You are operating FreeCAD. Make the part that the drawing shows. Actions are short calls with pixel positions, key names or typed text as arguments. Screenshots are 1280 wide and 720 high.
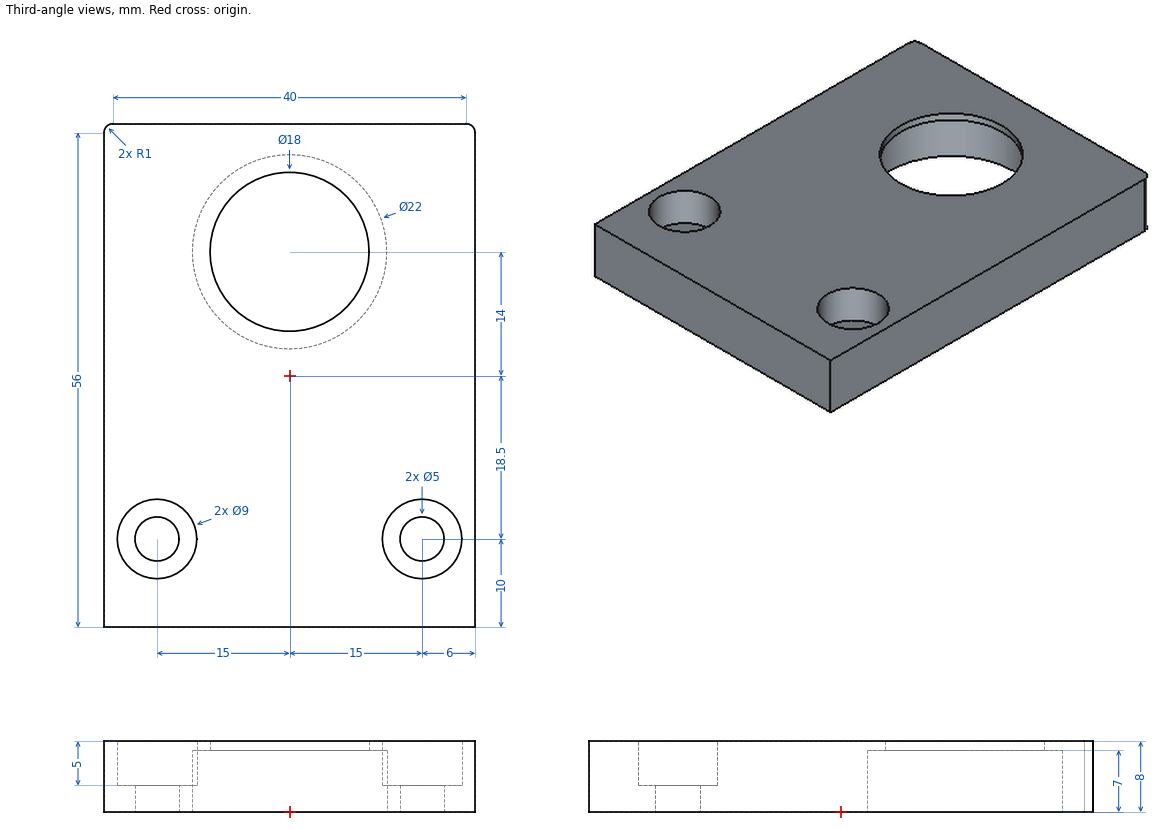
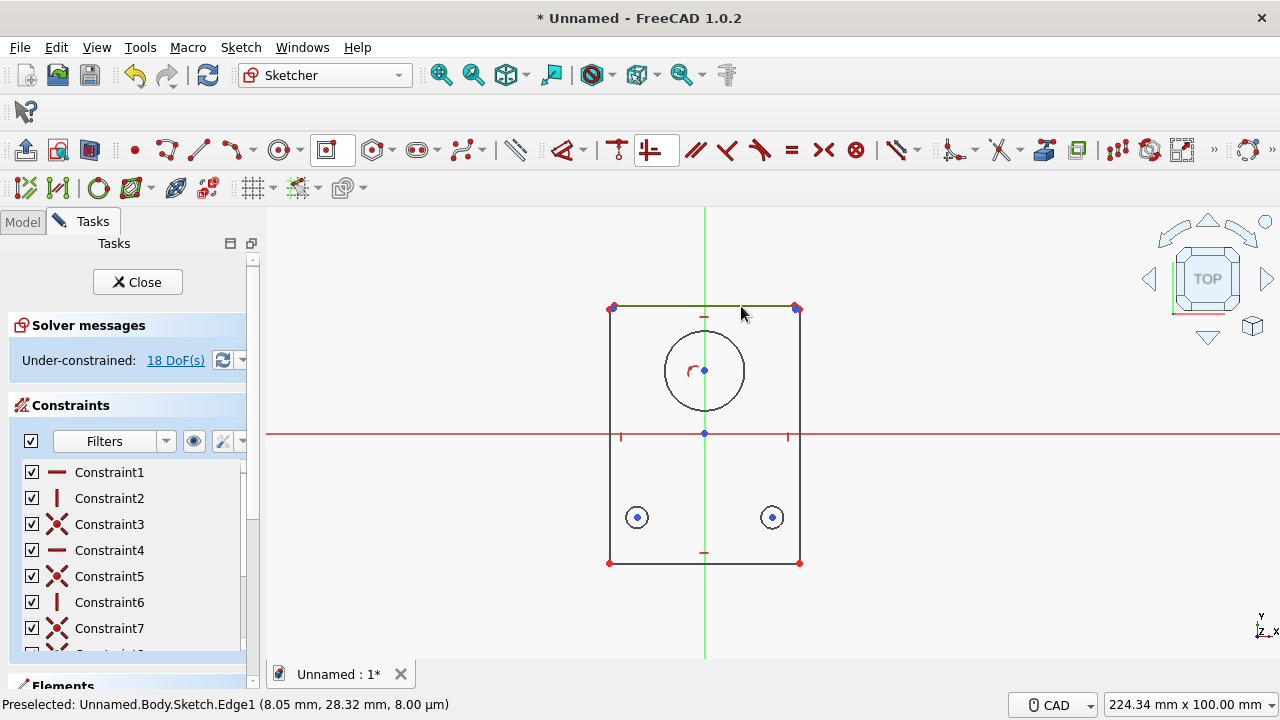
scroll(611, 306, up, 7)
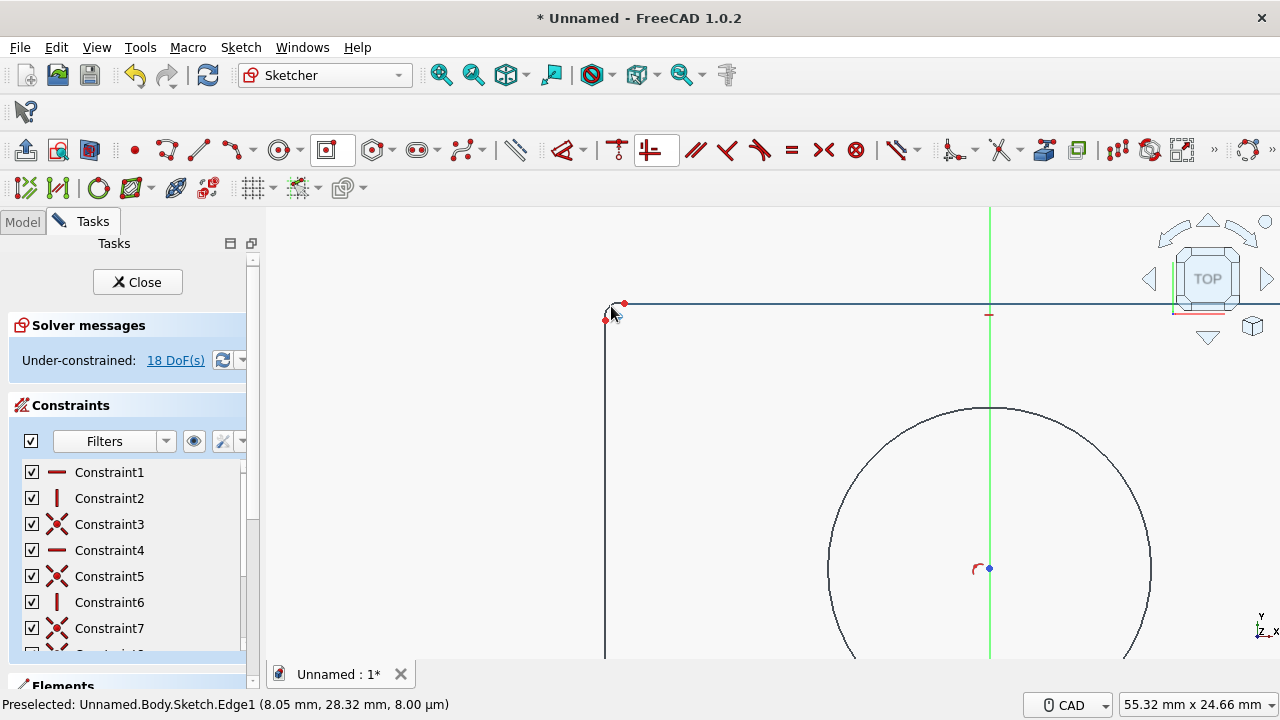
click(610, 306)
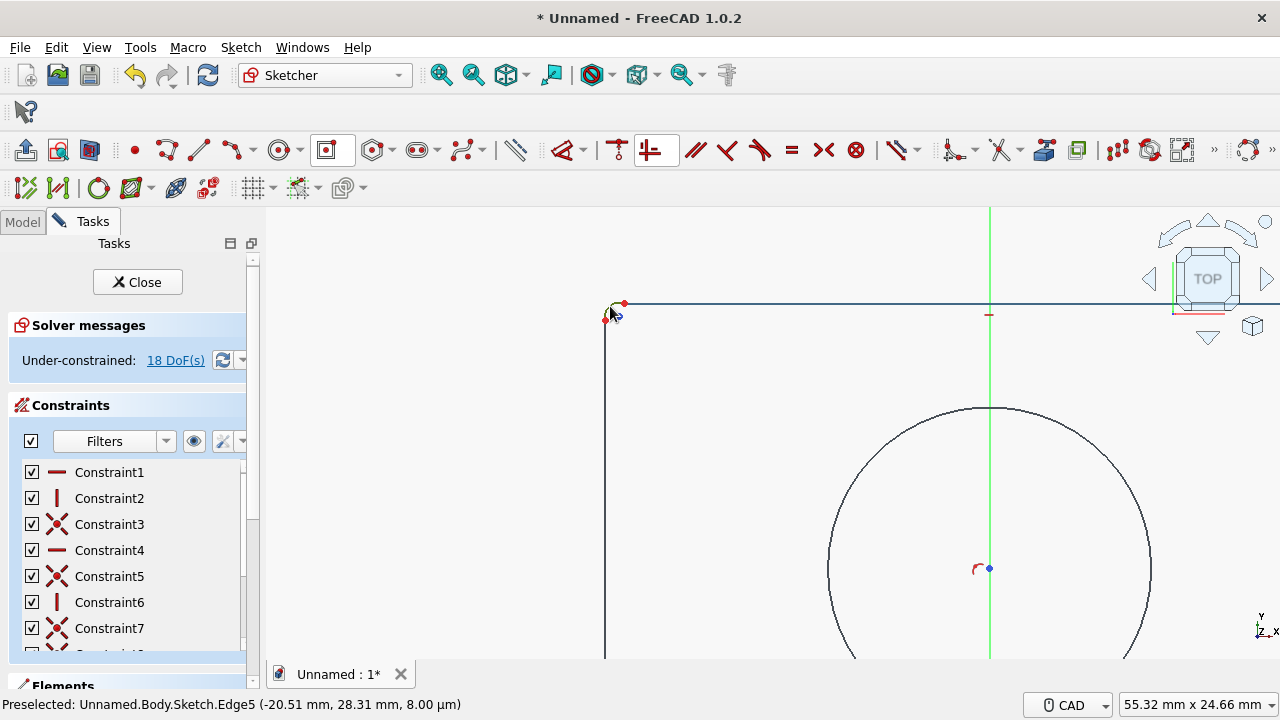
click(760, 150)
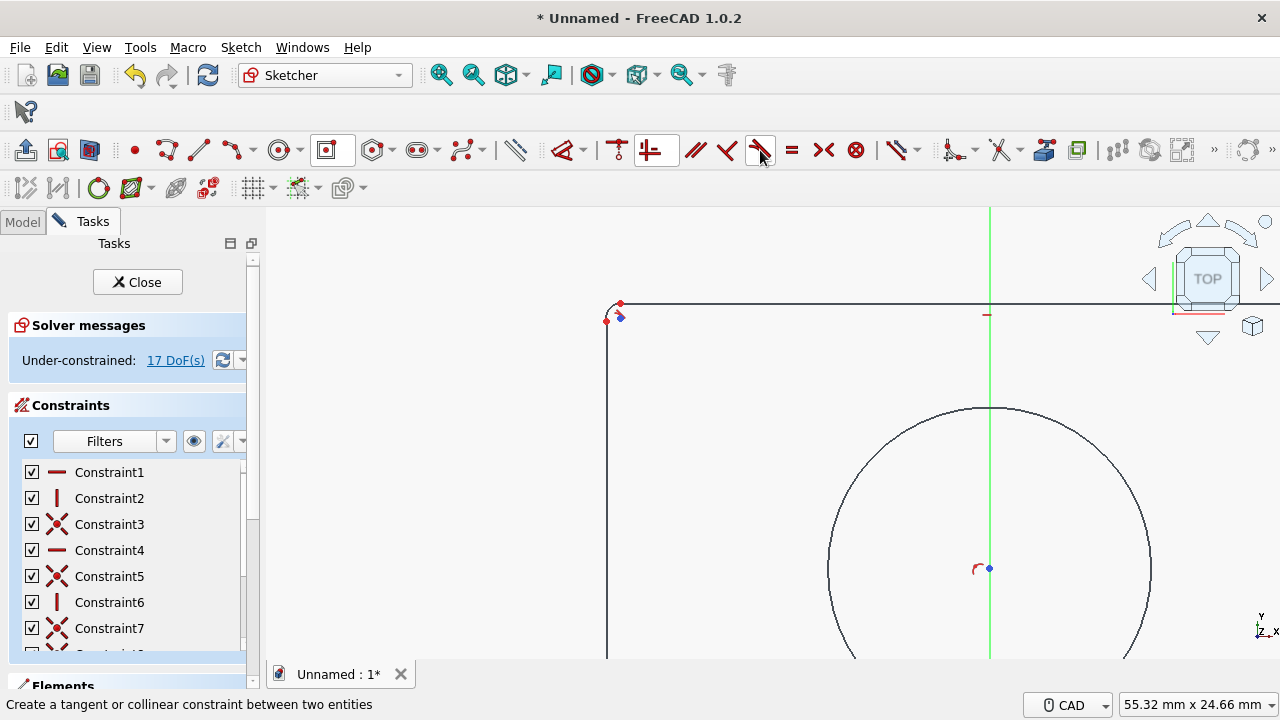
scroll(611, 305, down, 7)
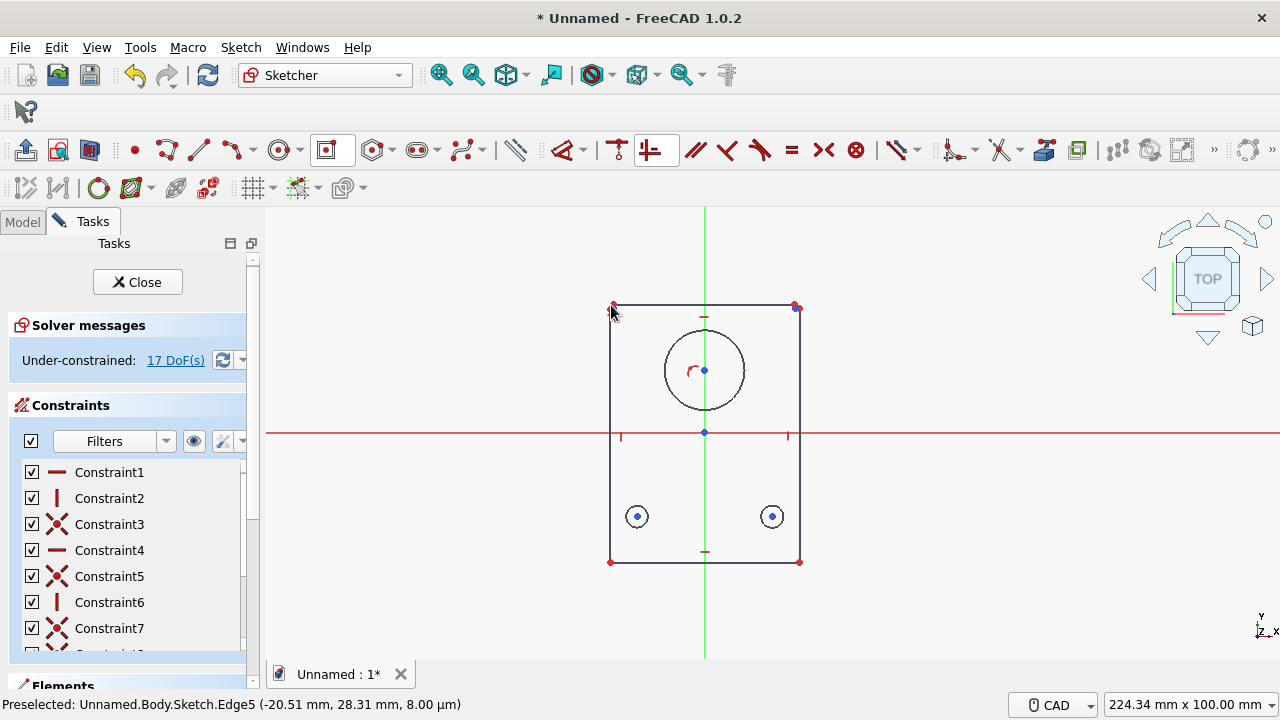
click(668, 305)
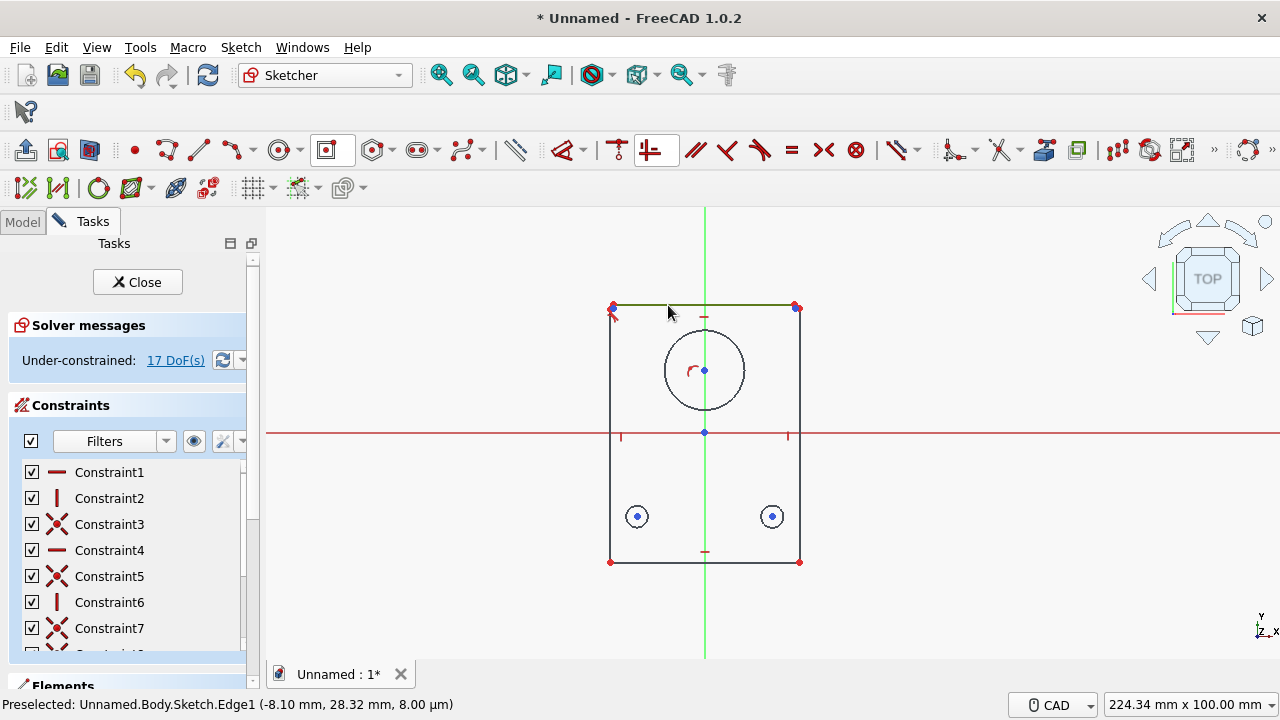
scroll(798, 306, up, 7)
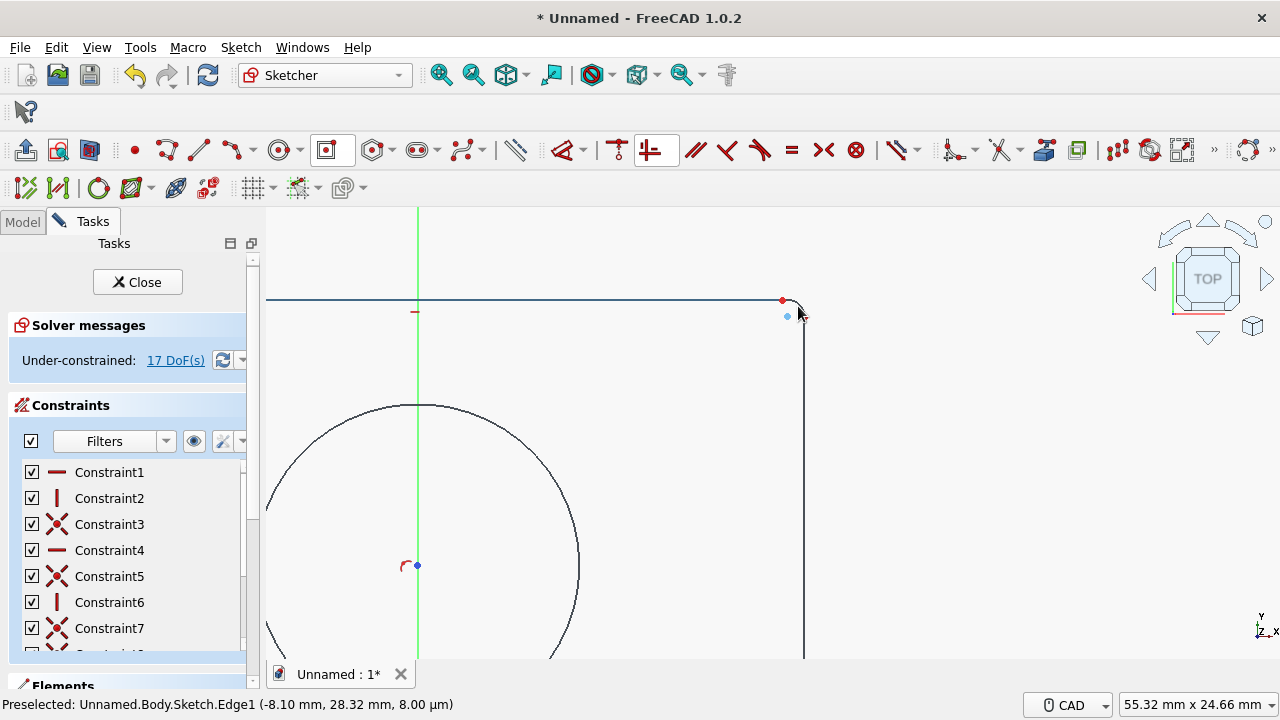
click(798, 303)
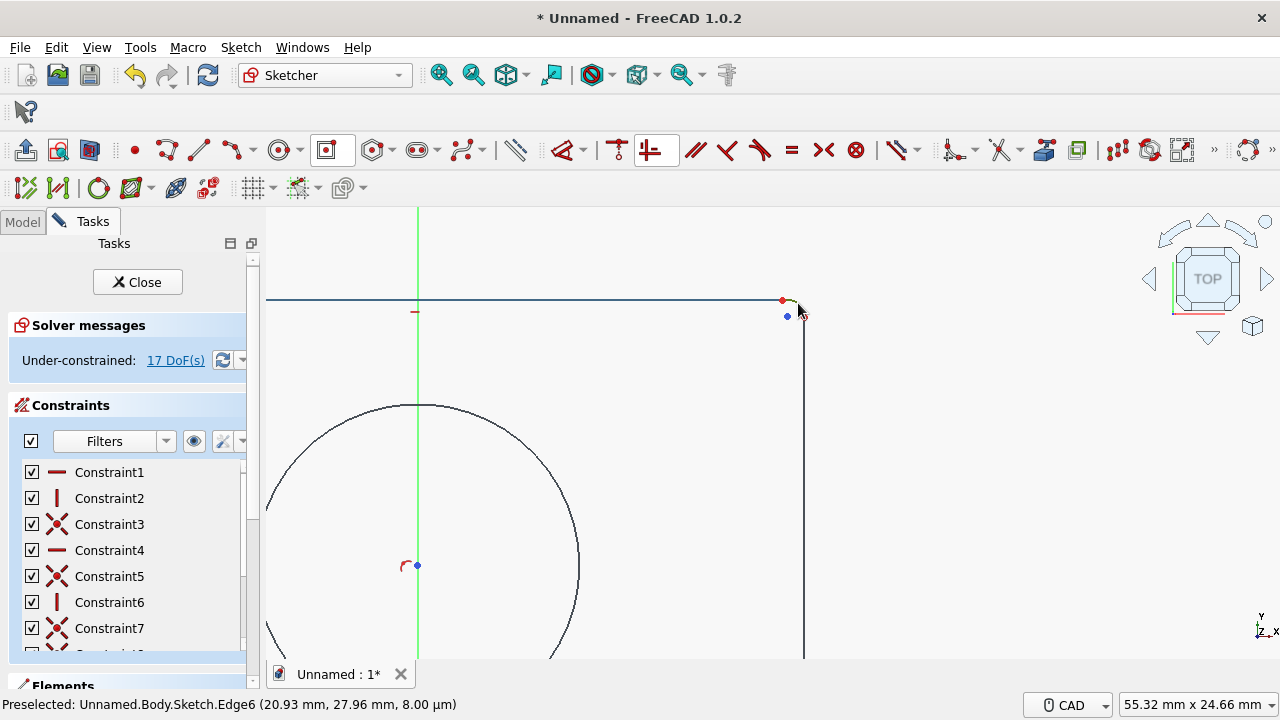
click(760, 150)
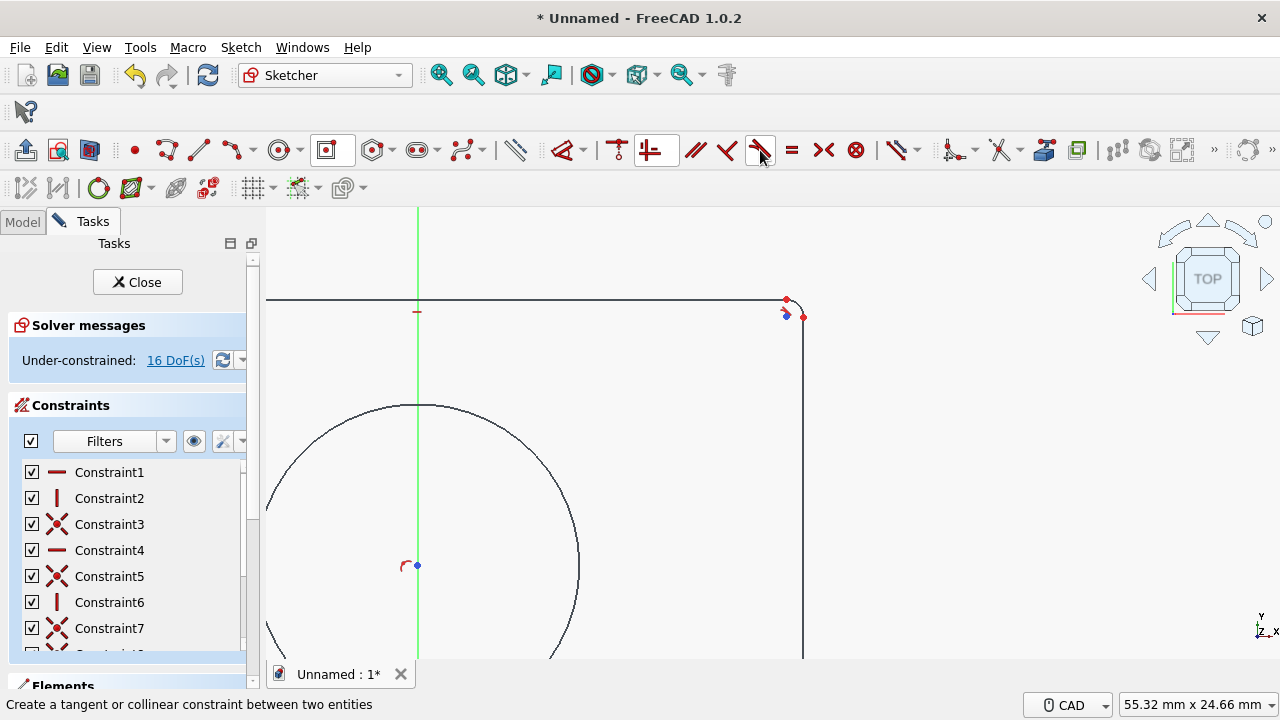
scroll(798, 306, down, 7)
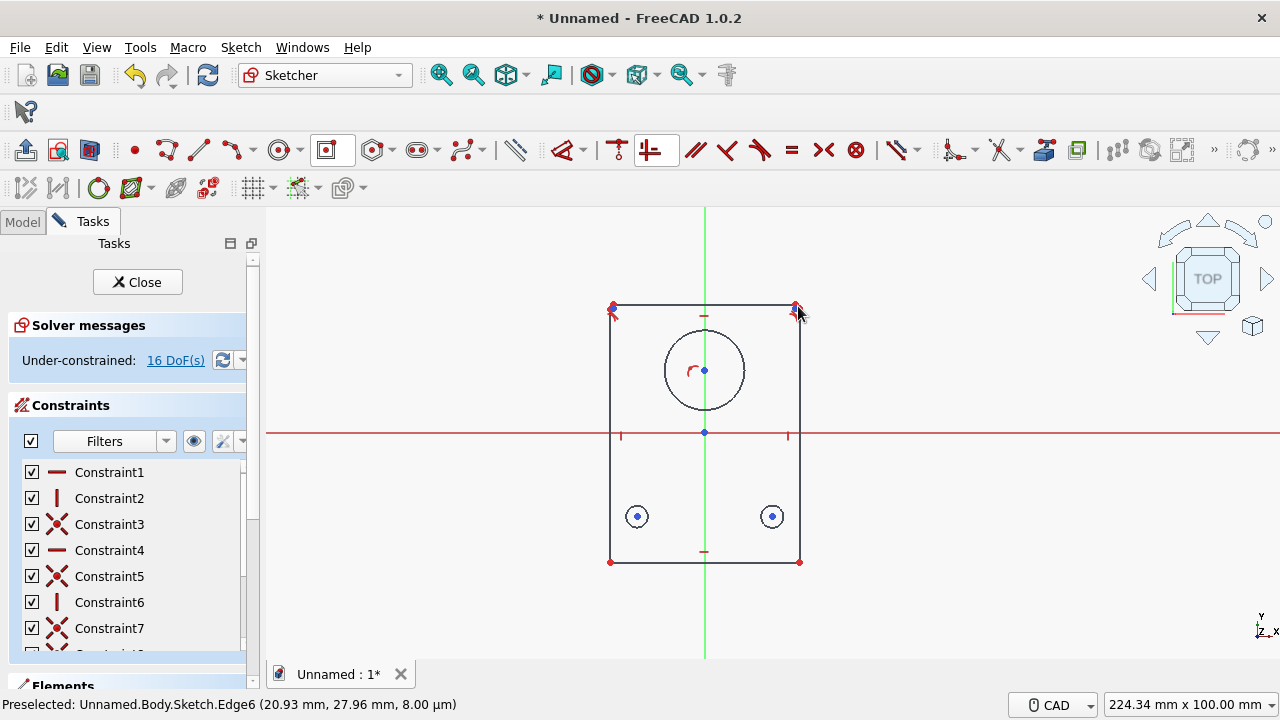
click(610, 385)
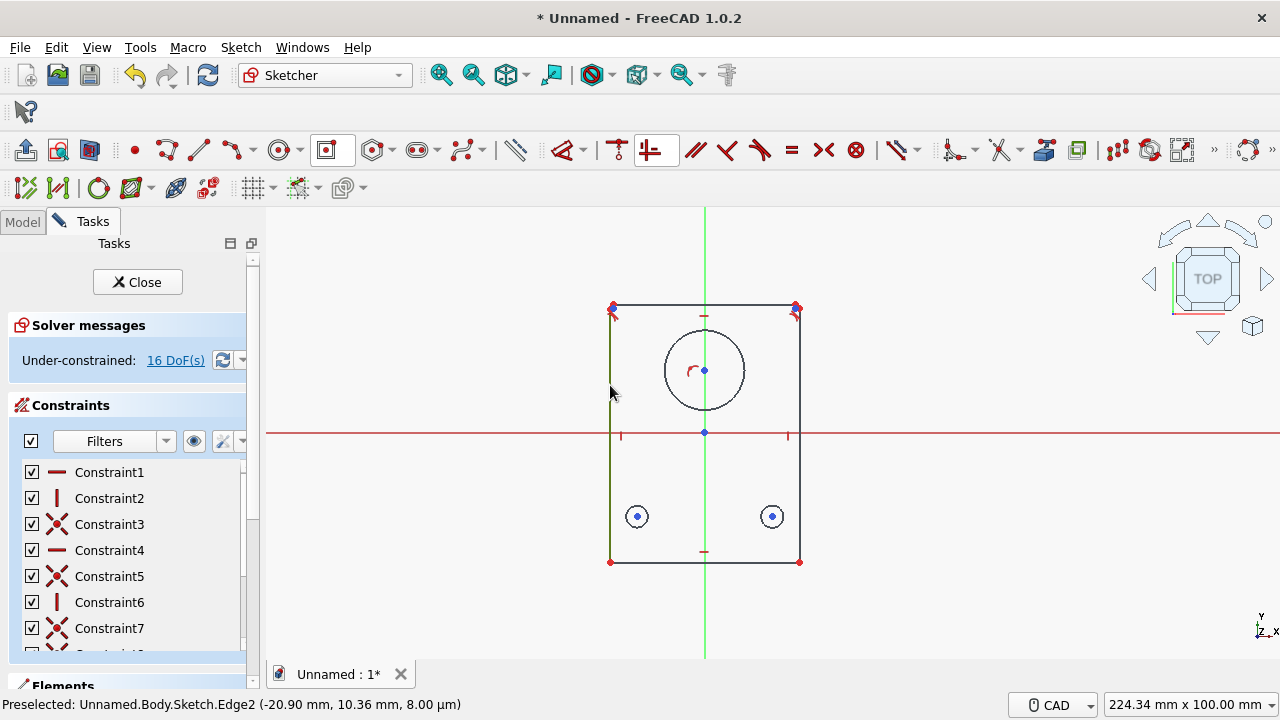
scroll(611, 306, up, 8)